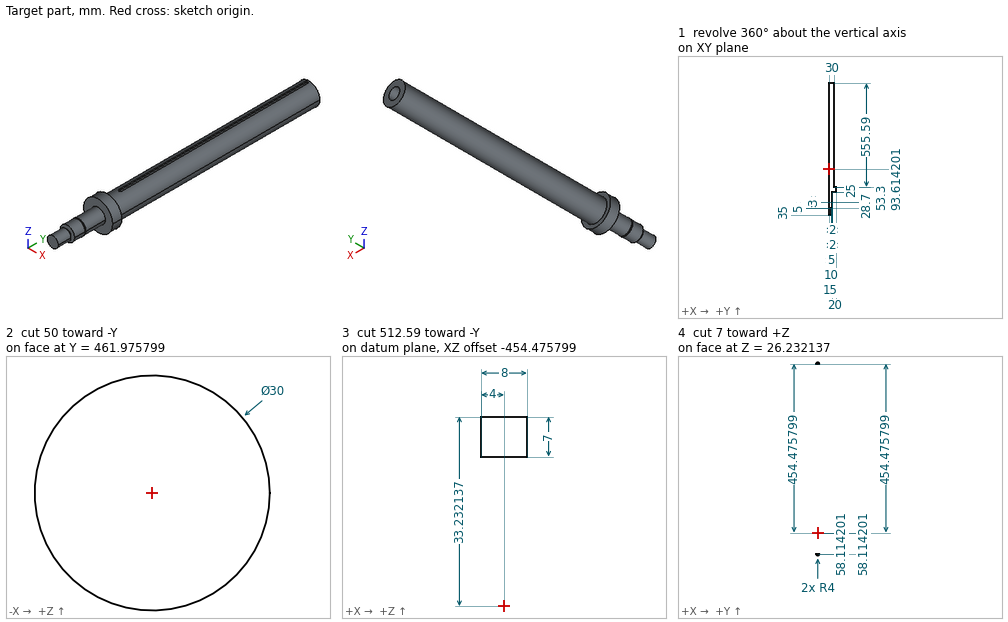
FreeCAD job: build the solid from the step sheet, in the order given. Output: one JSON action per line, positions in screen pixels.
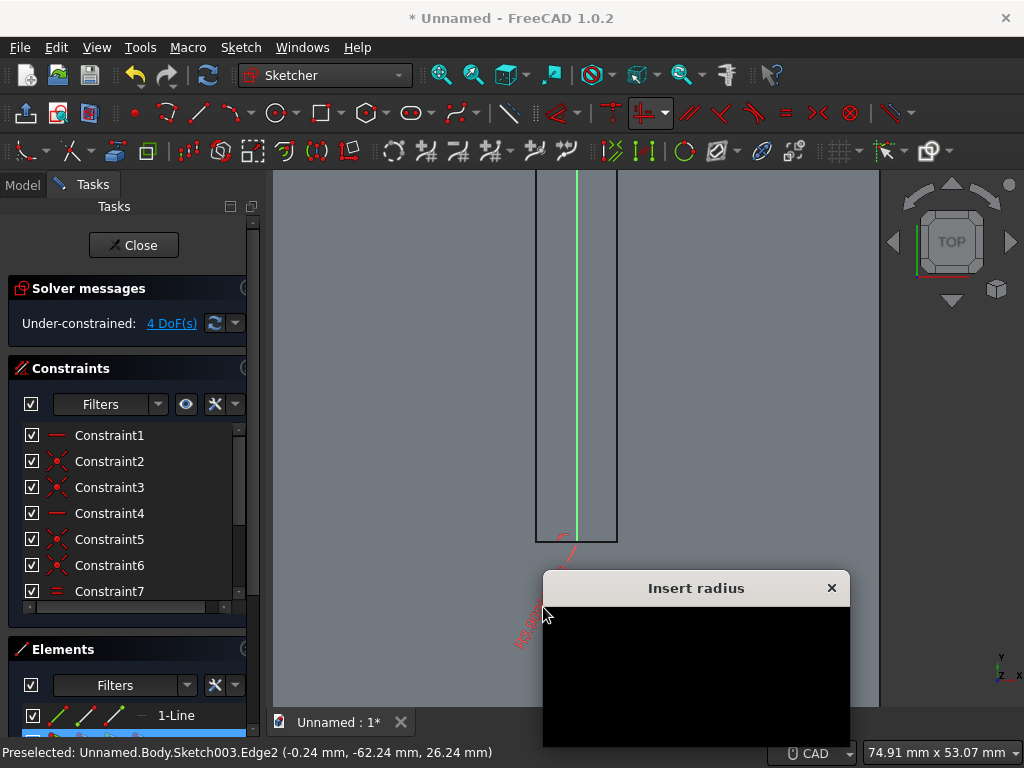
{"action": "type", "text": "4"}
{"action": "key", "text": "Return"}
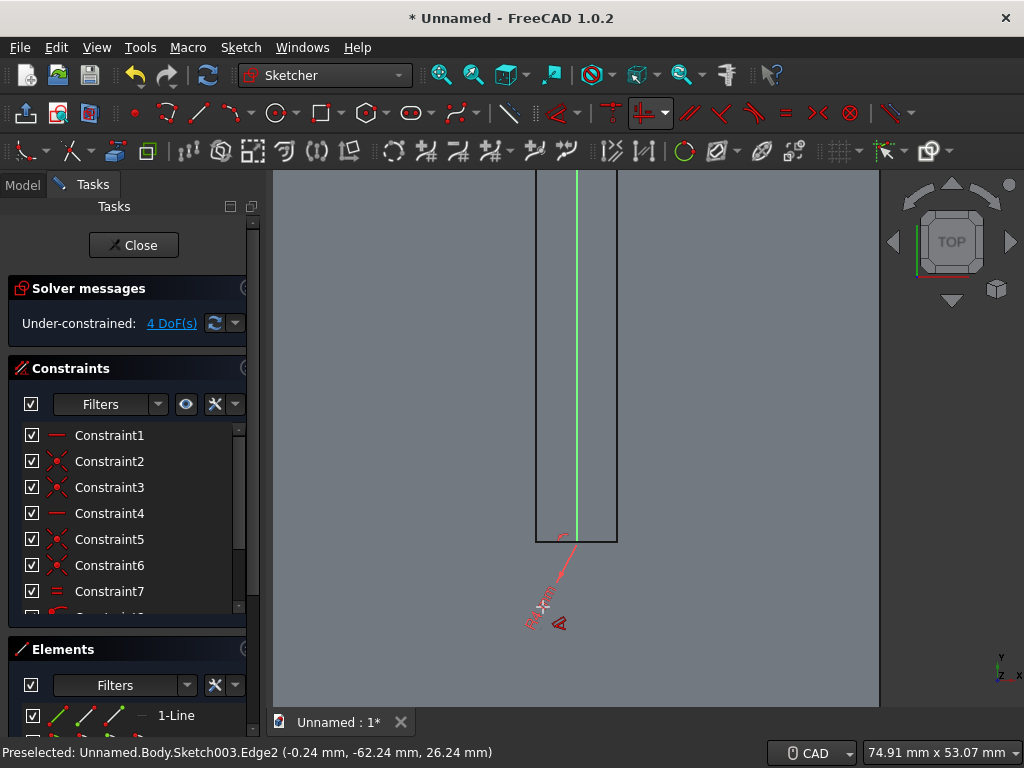
{"action": "scroll", "coordinate": [576, 600], "scroll_direction": "down", "scroll_amount": 14}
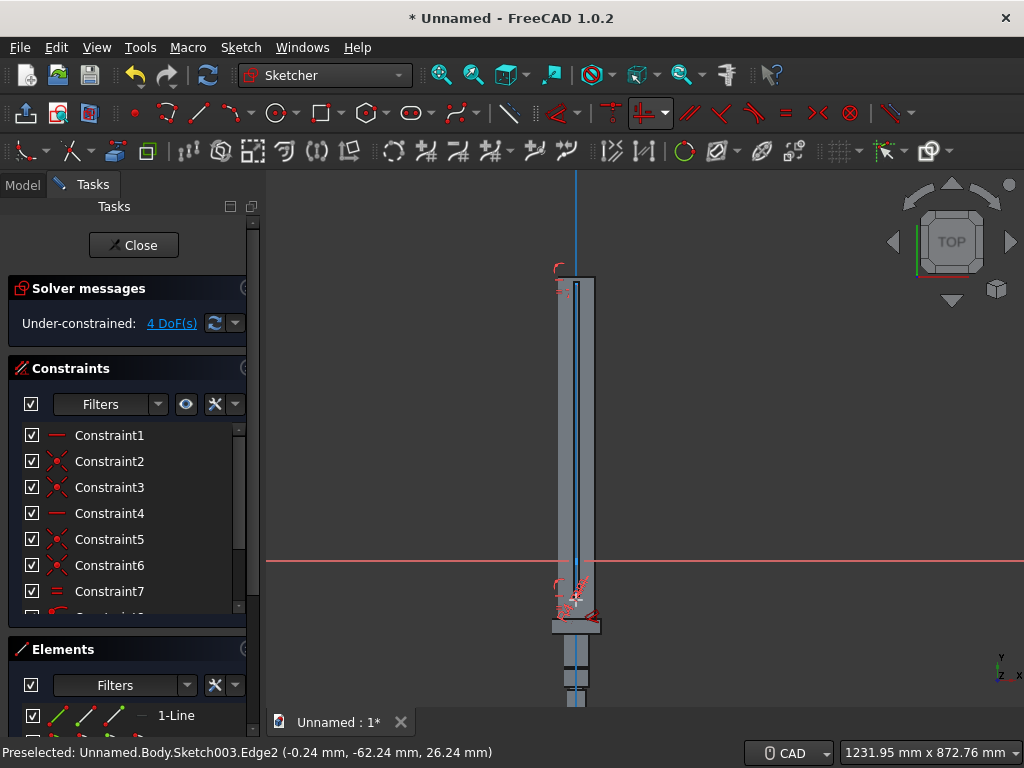
{"action": "scroll", "coordinate": [579, 597], "scroll_direction": "up", "scroll_amount": 9}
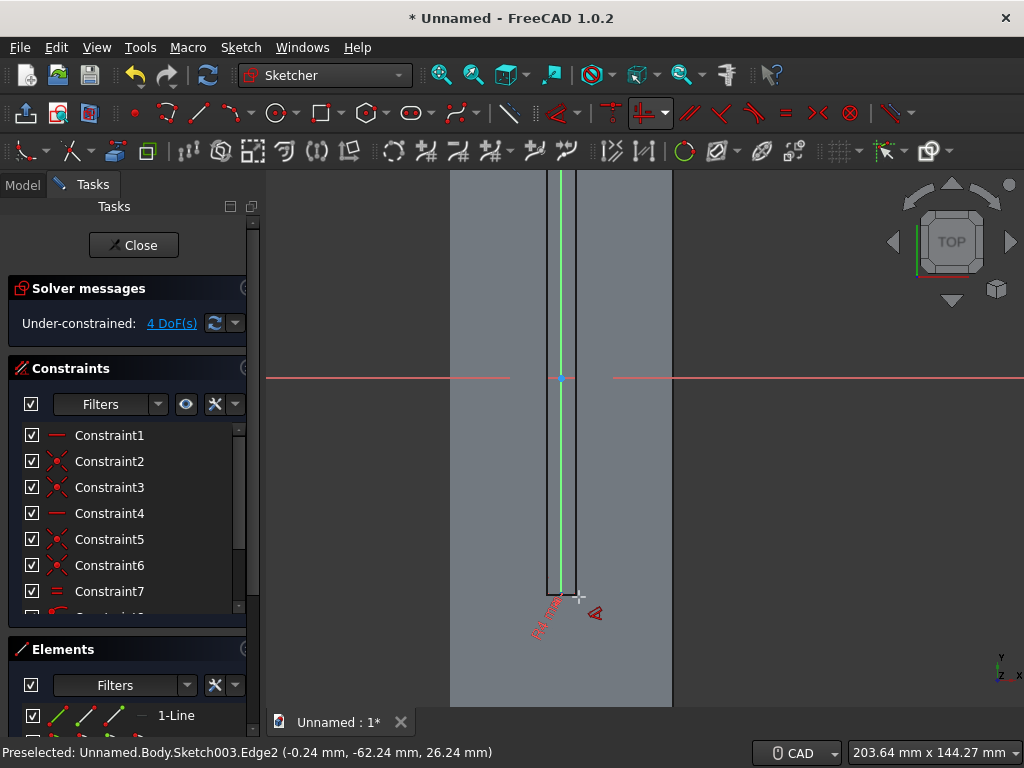
{"action": "left_click", "coordinate": [576, 595]}
{"action": "left_click", "coordinate": [610, 487]}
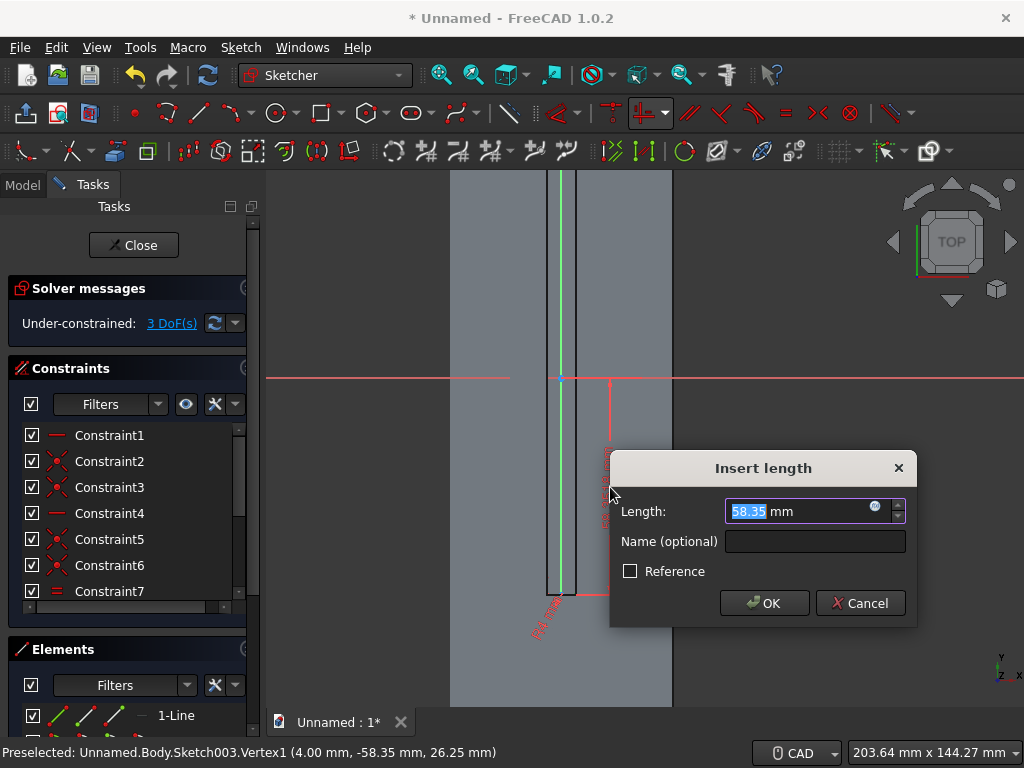
{"action": "type", "text": "58.114201"}
{"action": "key", "text": "Return"}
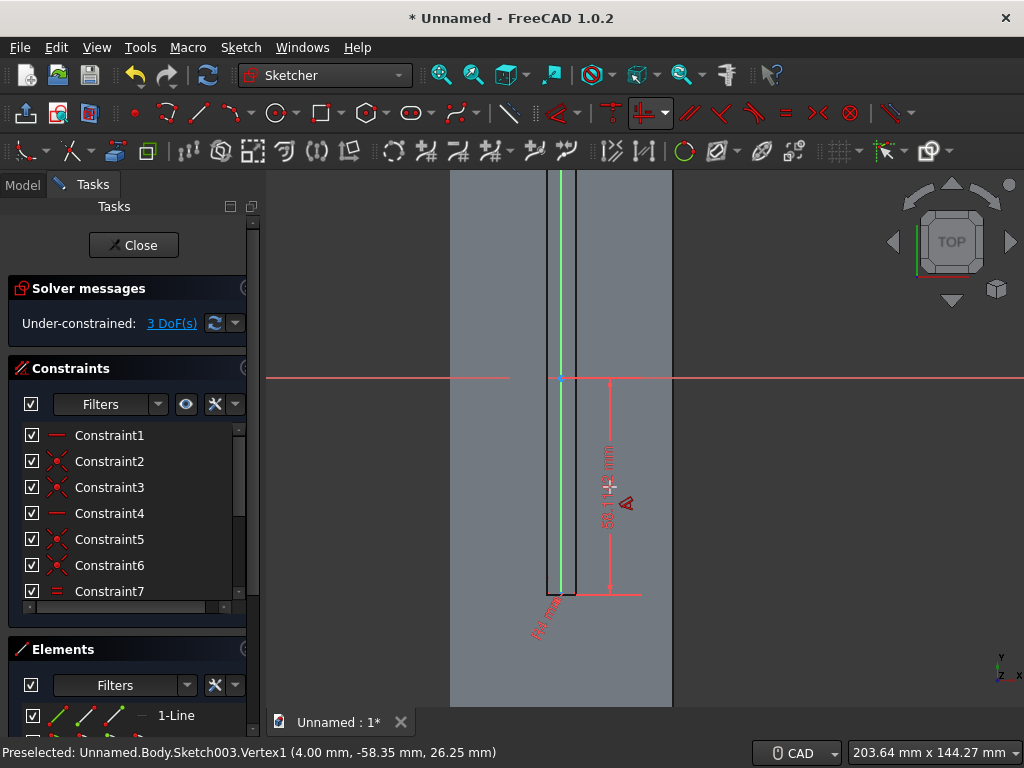
{"action": "left_click", "coordinate": [561, 595]}
{"action": "left_click", "coordinate": [595, 437]}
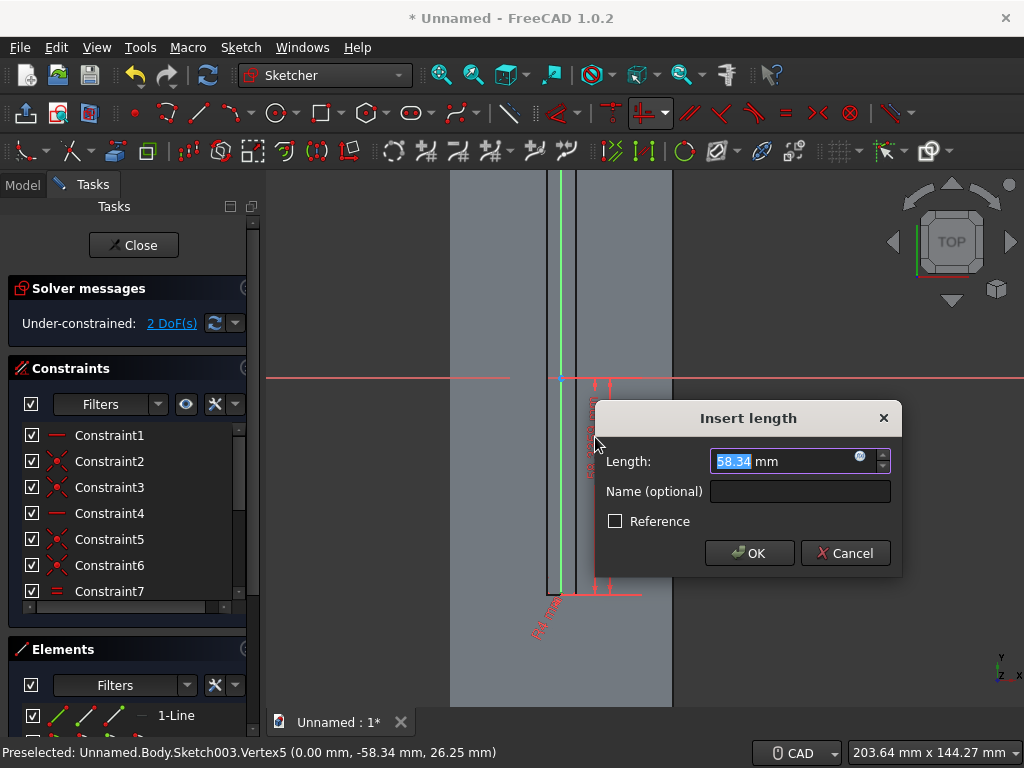
{"action": "type", "text": "58.114201"}
{"action": "key", "text": "Return"}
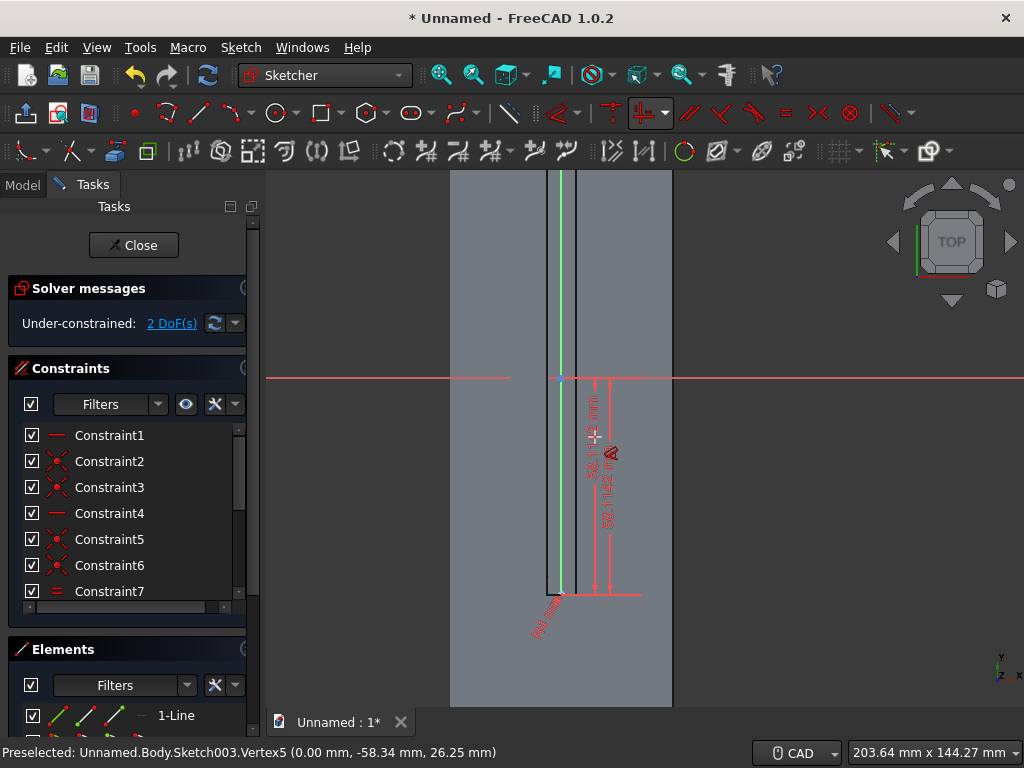
{"action": "scroll", "coordinate": [579, 597], "scroll_direction": "down", "scroll_amount": 9}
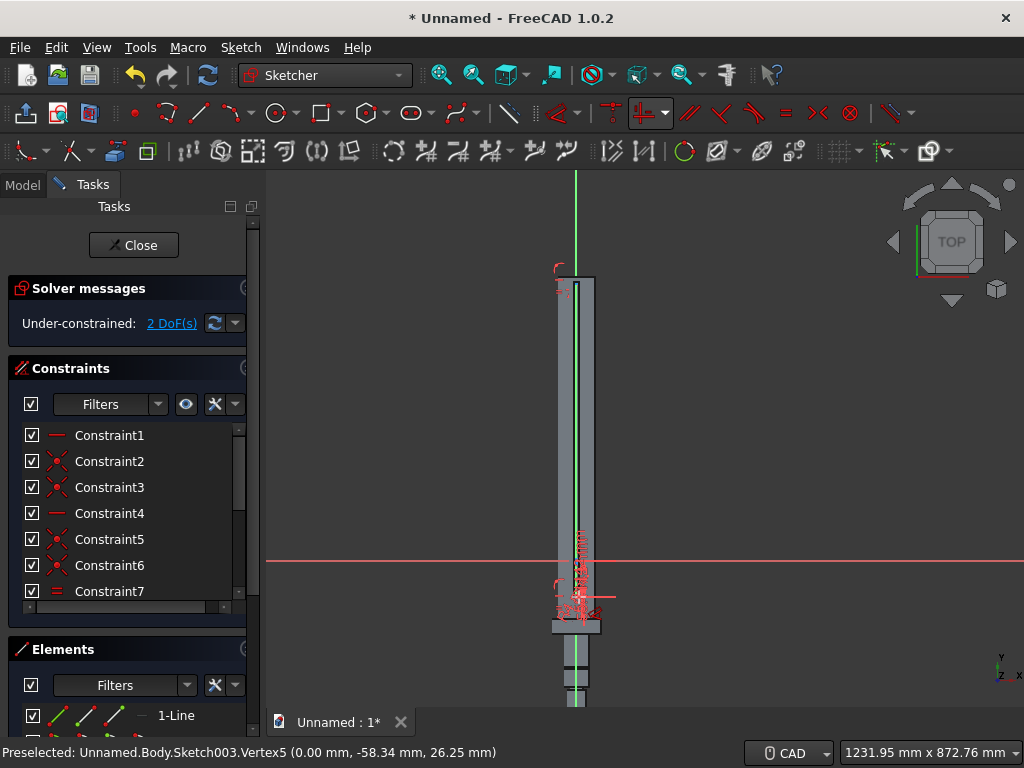
{"action": "scroll", "coordinate": [574, 282], "scroll_direction": "up", "scroll_amount": 9}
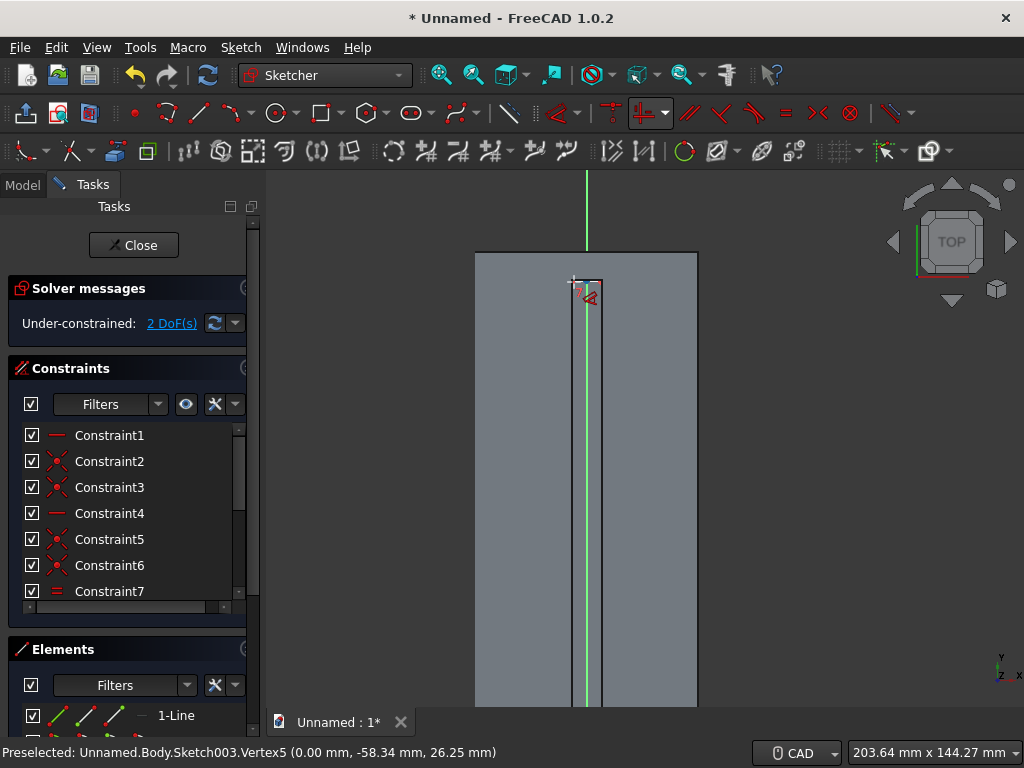
{"action": "left_click", "coordinate": [572, 281]}
{"action": "left_click", "coordinate": [538, 480]}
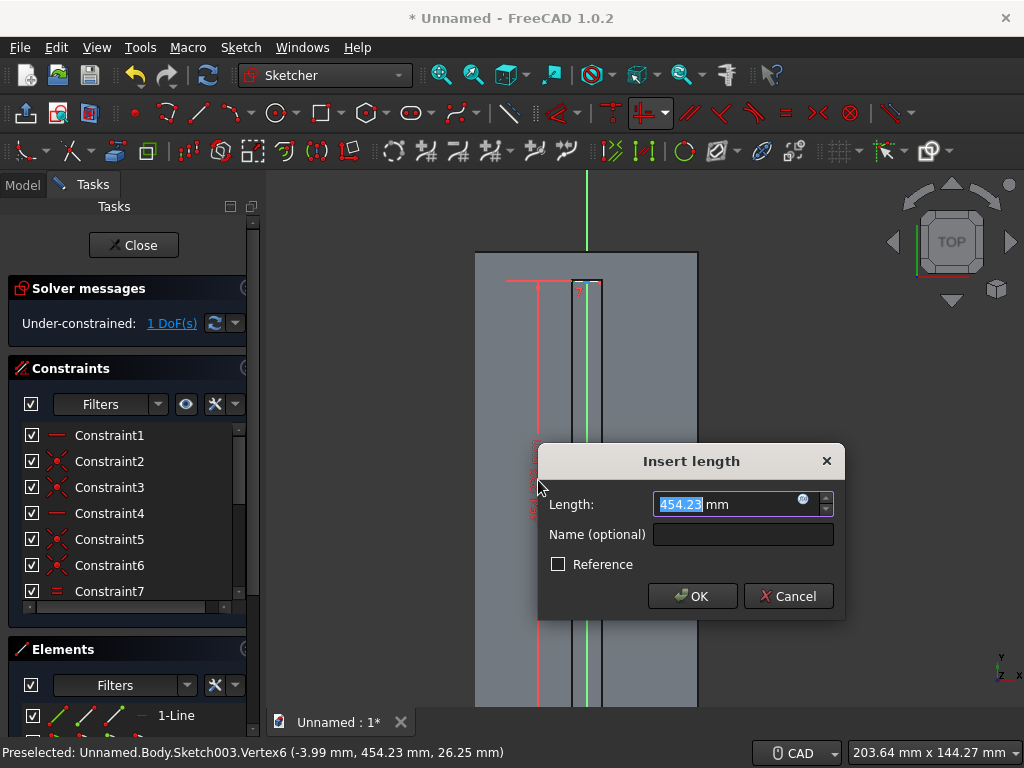
{"action": "type", "text": "454.475799"}
{"action": "key", "text": "Return"}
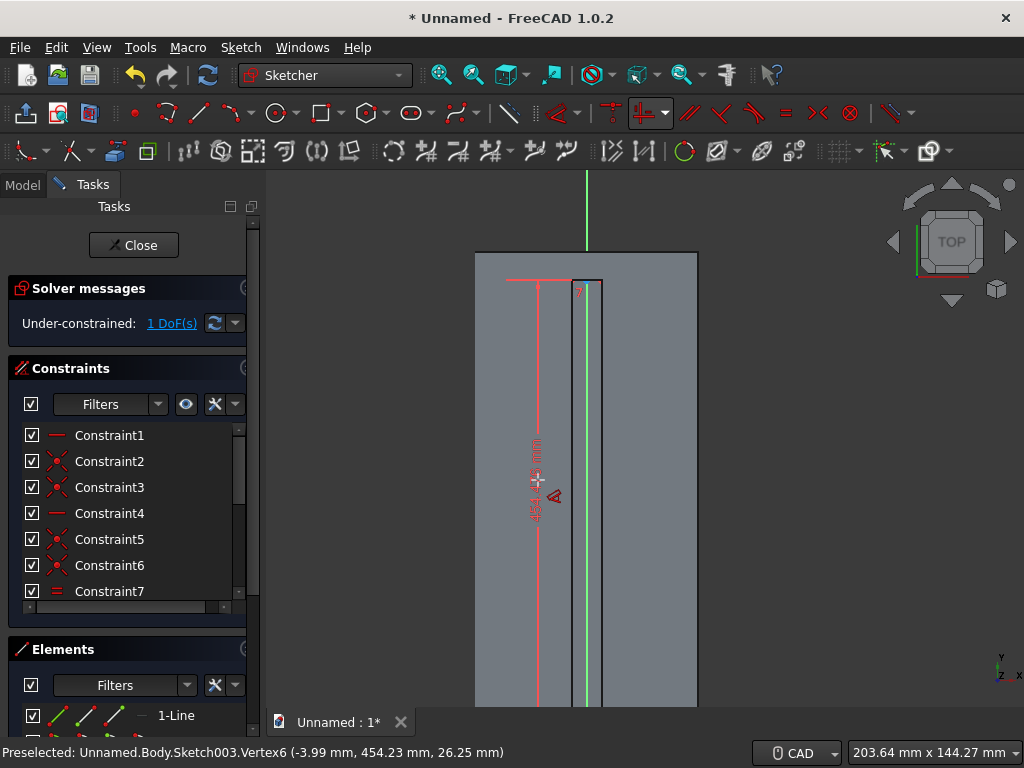
{"action": "left_click", "coordinate": [587, 280]}
{"action": "left_click", "coordinate": [621, 480]}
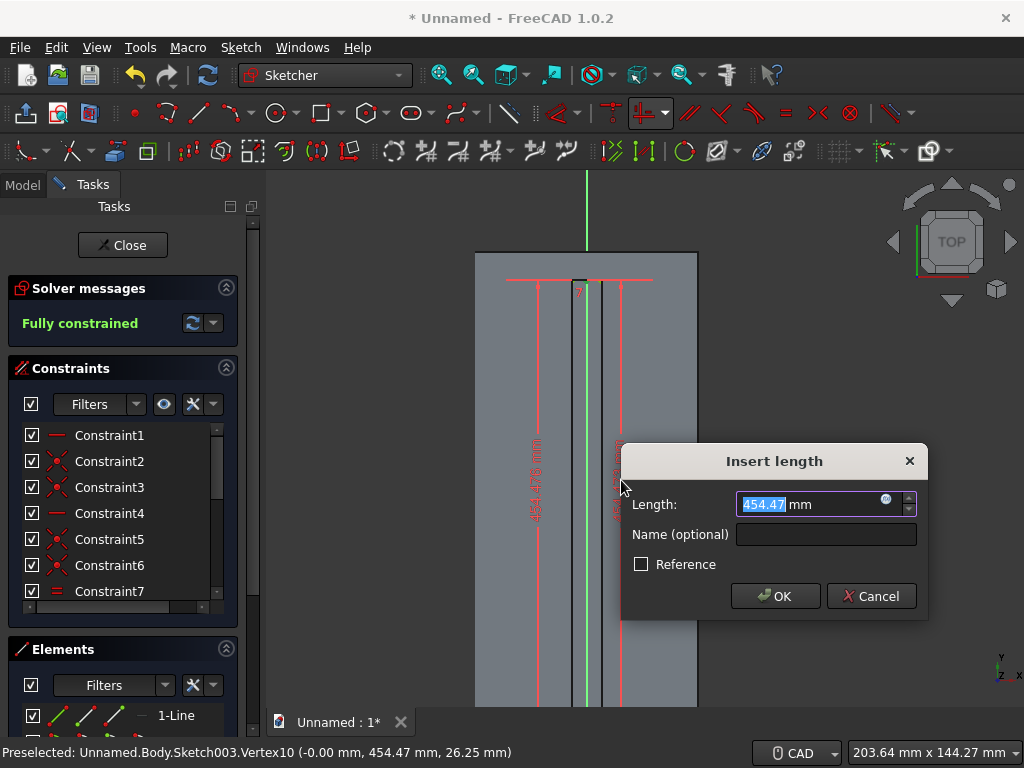
{"action": "type", "text": "454.475799"}
{"action": "key", "text": "Return"}
{"action": "key", "text": "Escape"}